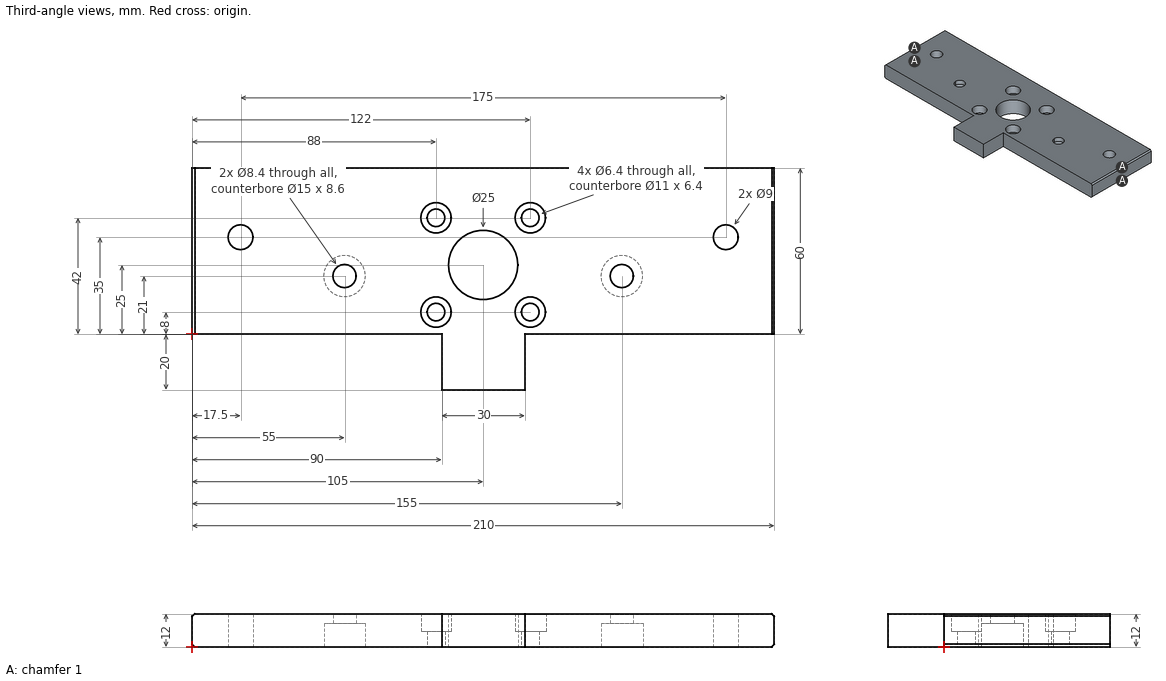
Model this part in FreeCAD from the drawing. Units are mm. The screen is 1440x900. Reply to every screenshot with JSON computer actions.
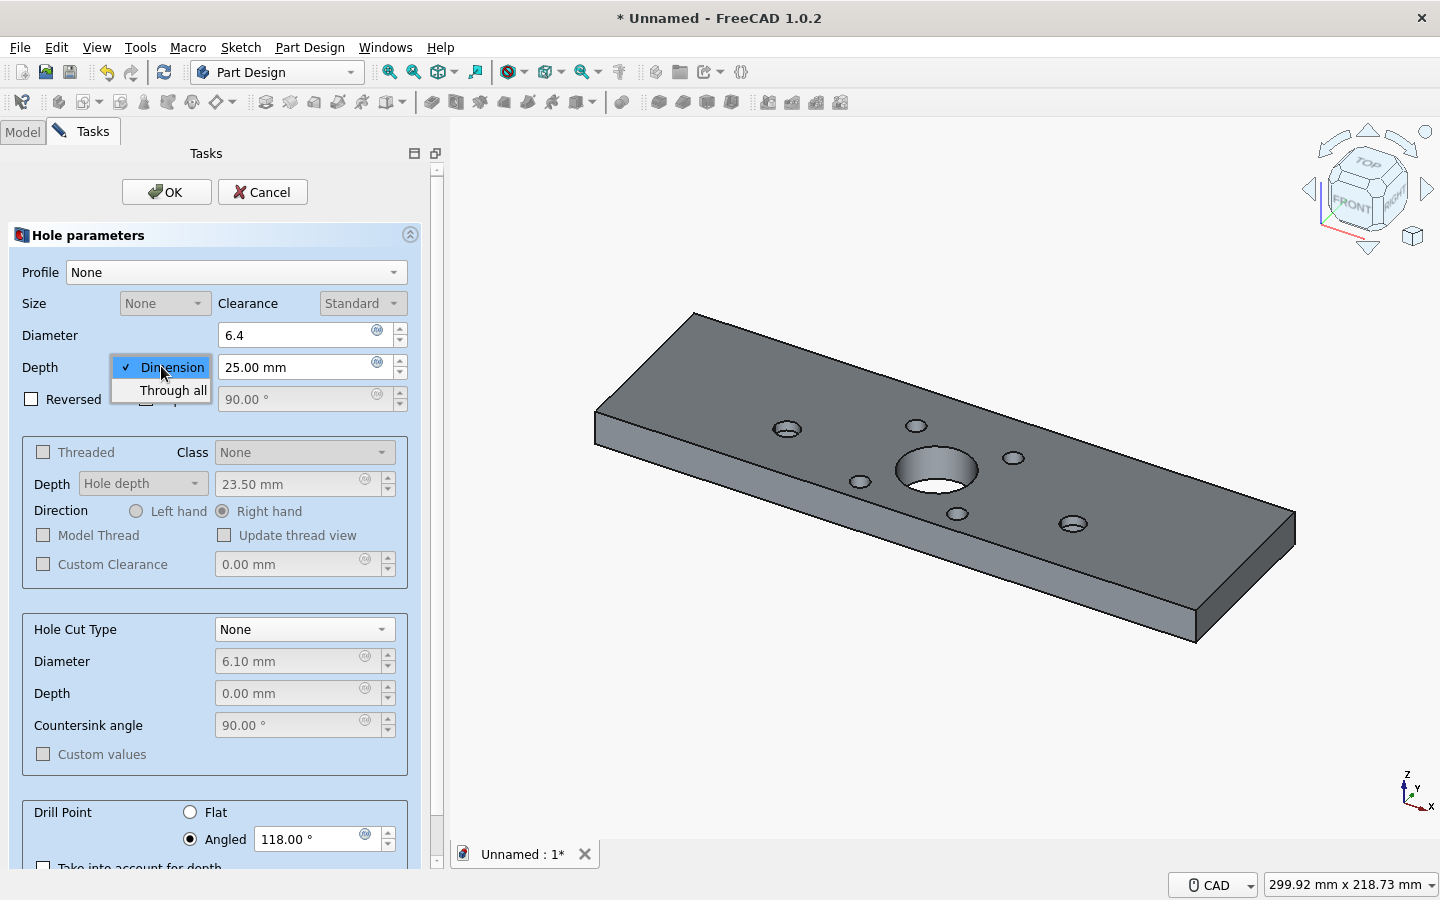
{"action": "left_click", "coordinate": [160, 390]}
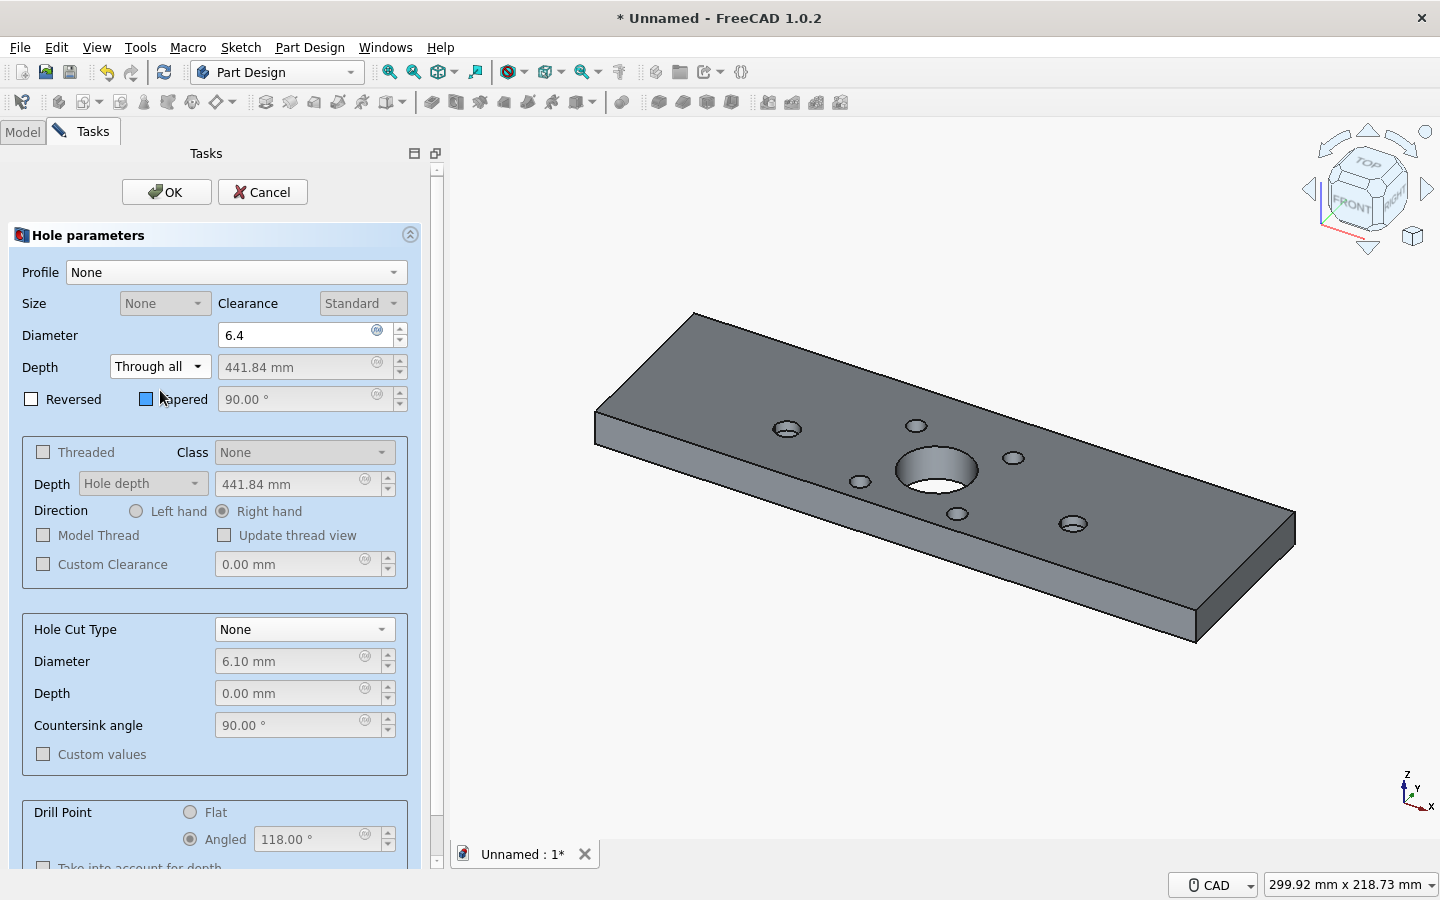
{"action": "left_click", "coordinate": [306, 630]}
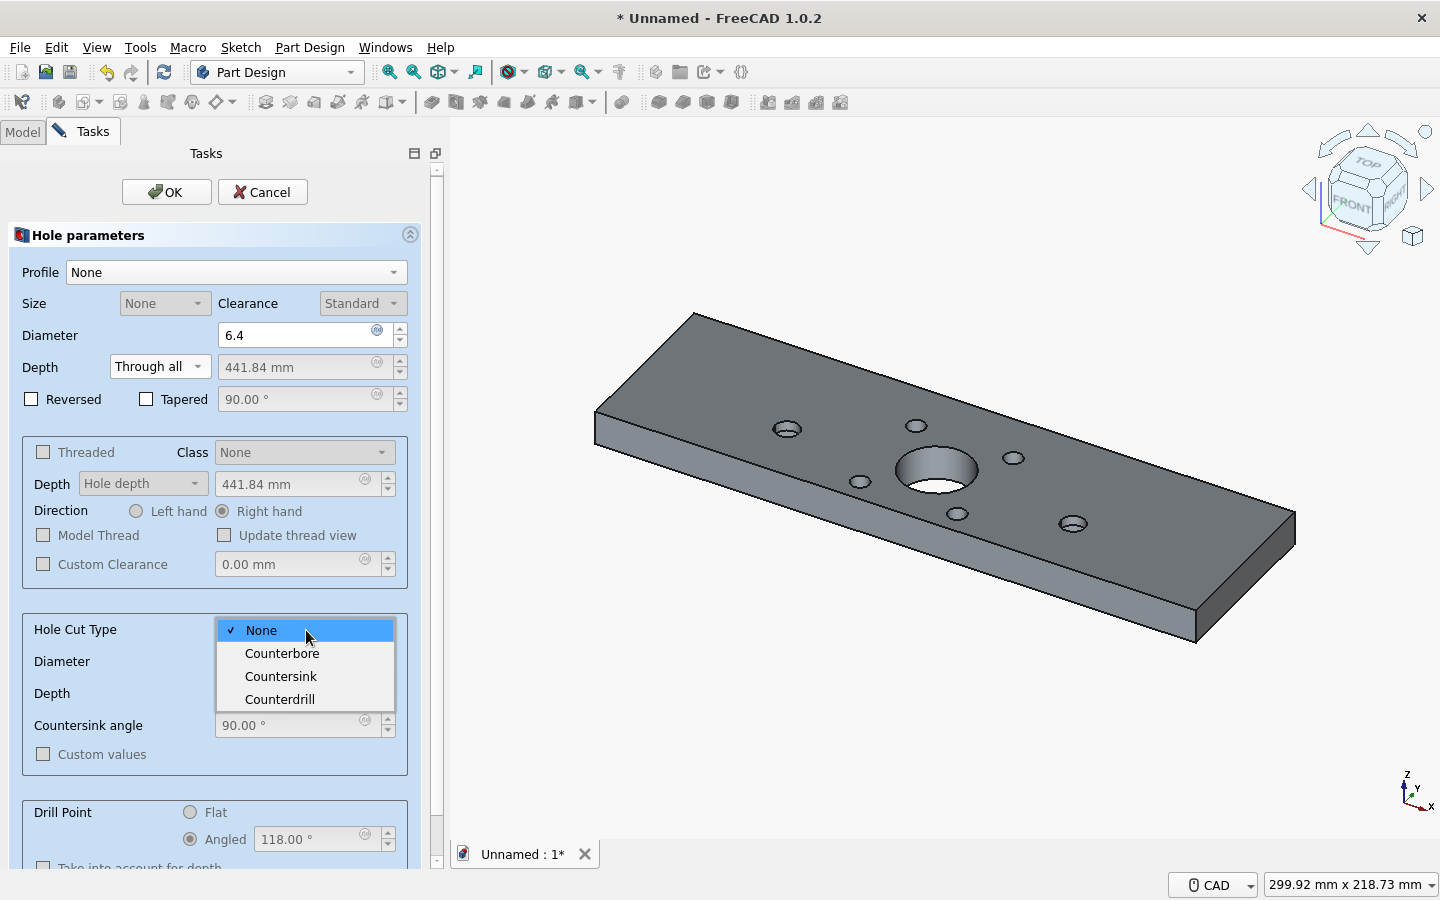
{"action": "left_click", "coordinate": [304, 654]}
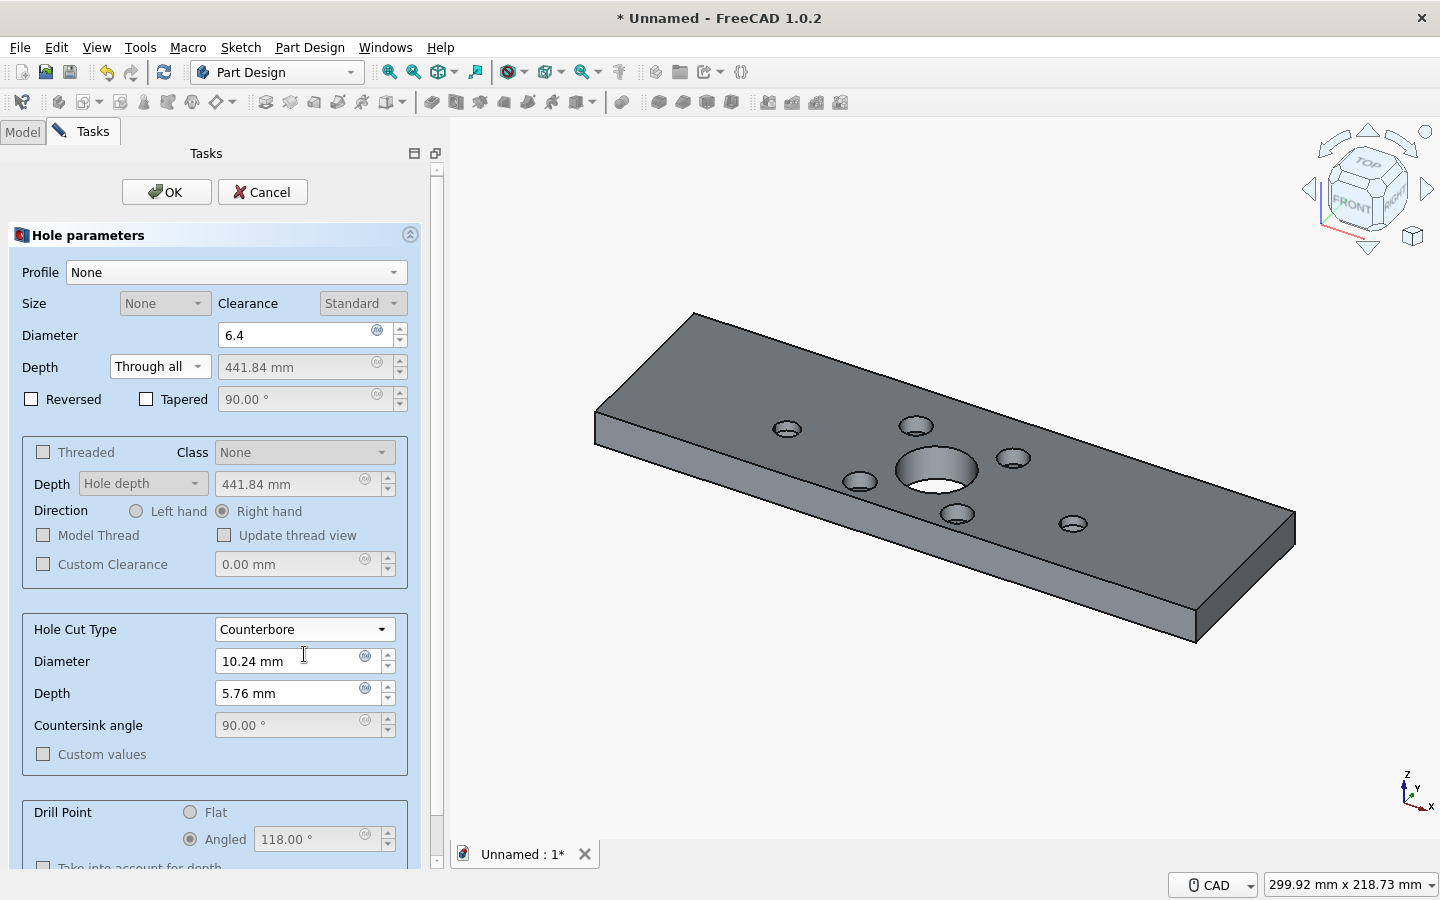
{"action": "triple_click", "coordinate": [298, 661]}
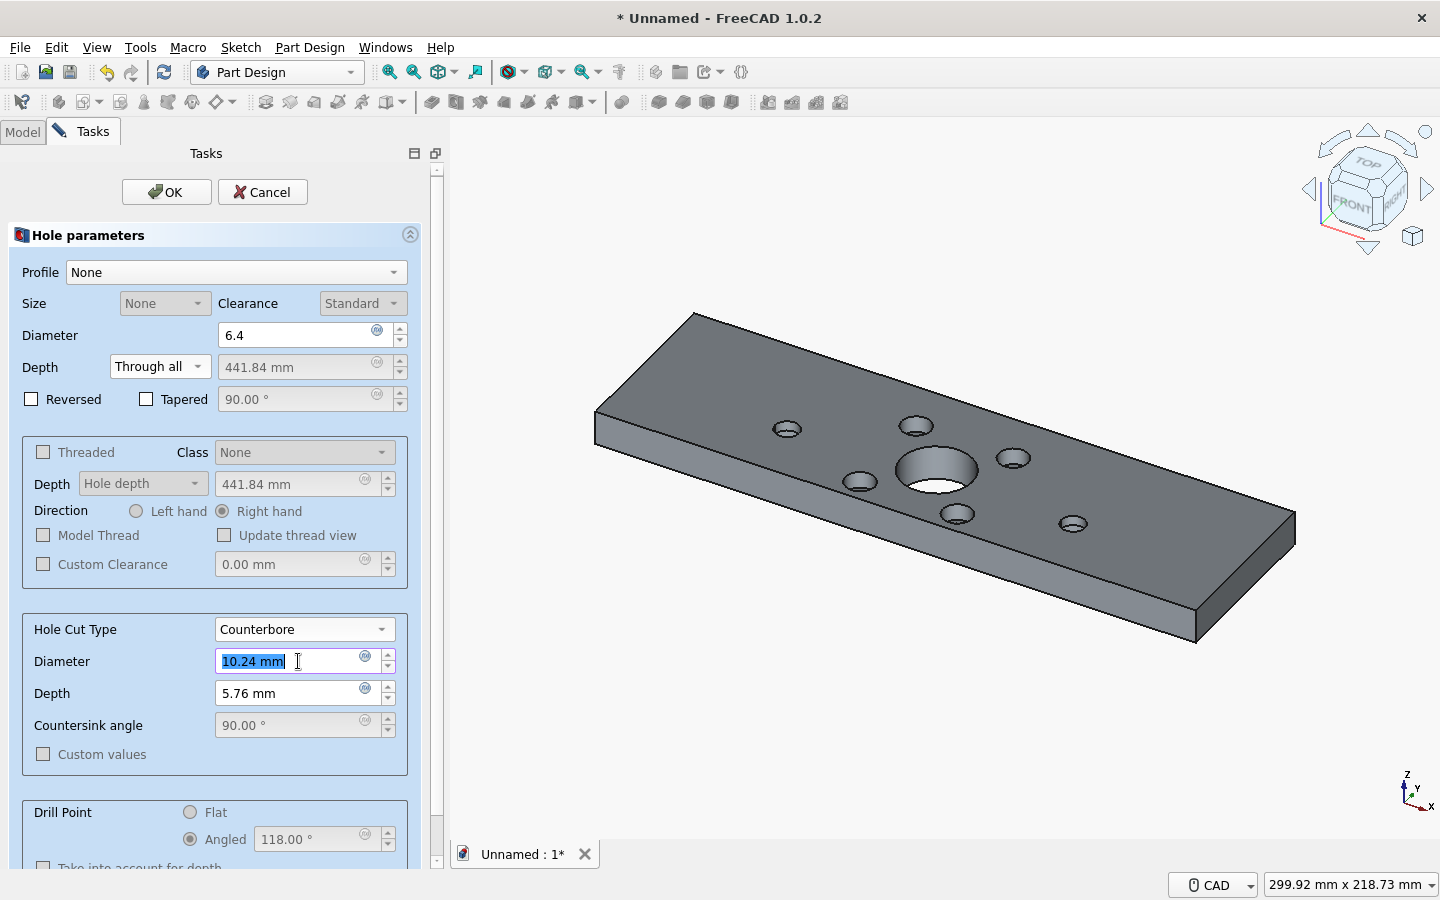
{"action": "type", "text": "11"}
{"action": "key", "text": "Tab"}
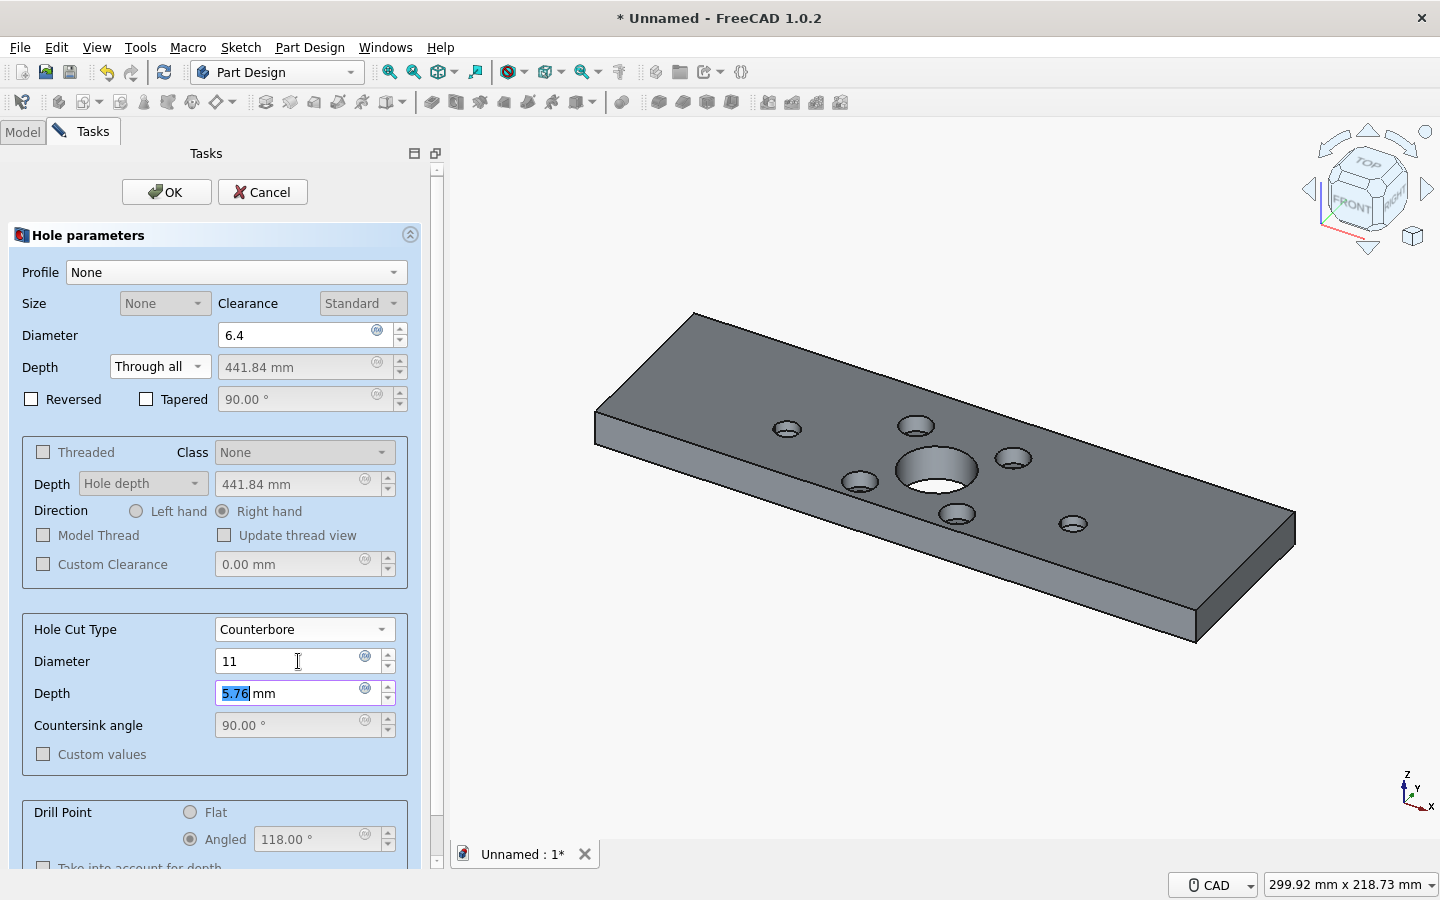
{"action": "type", "text": "6.4"}
{"action": "key", "text": "Tab"}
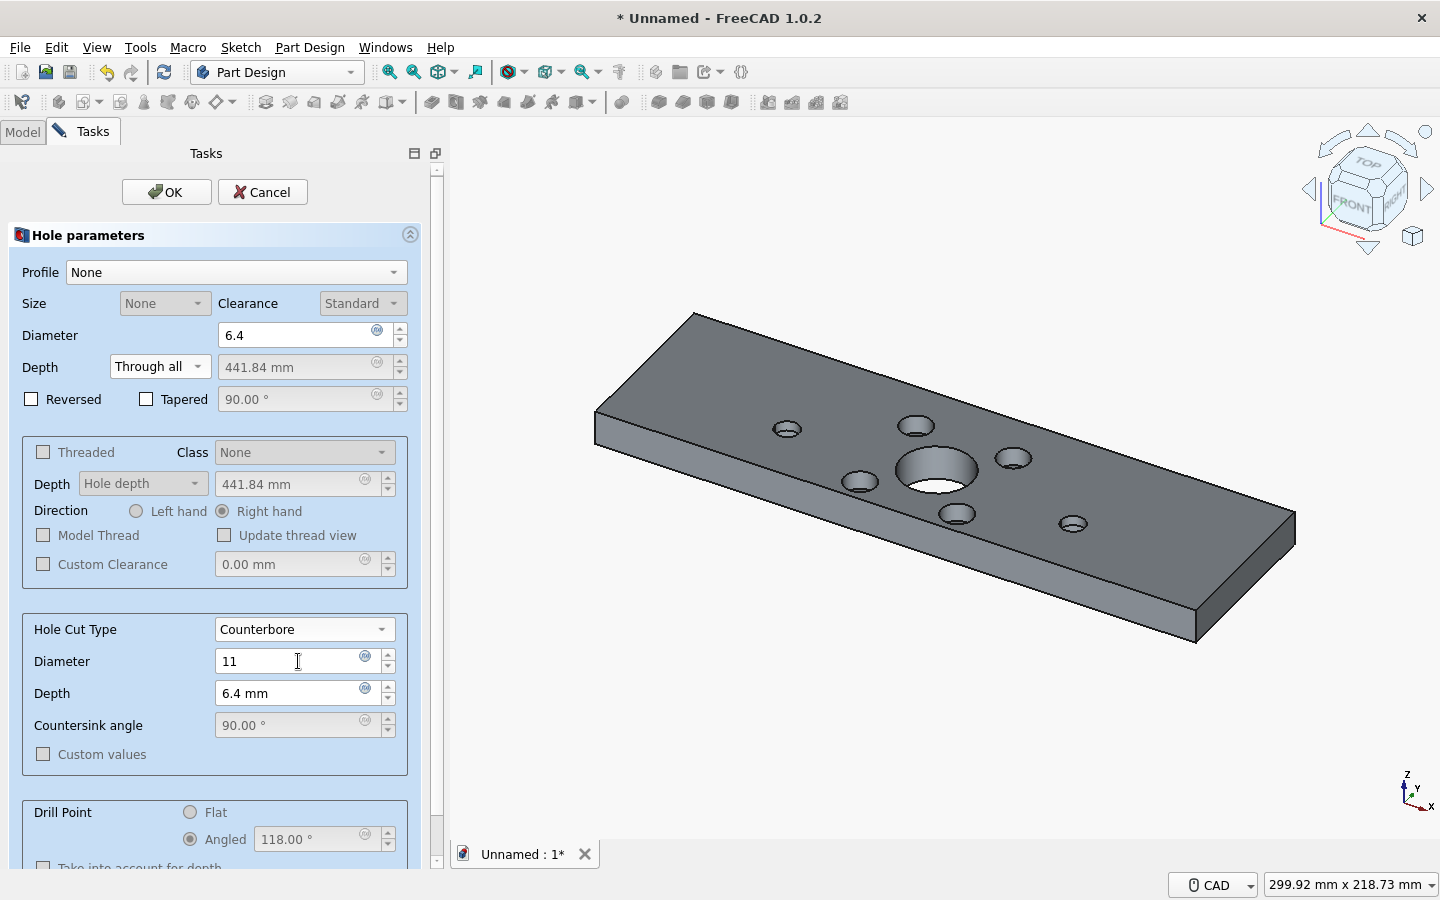
{"action": "left_click", "coordinate": [167, 192]}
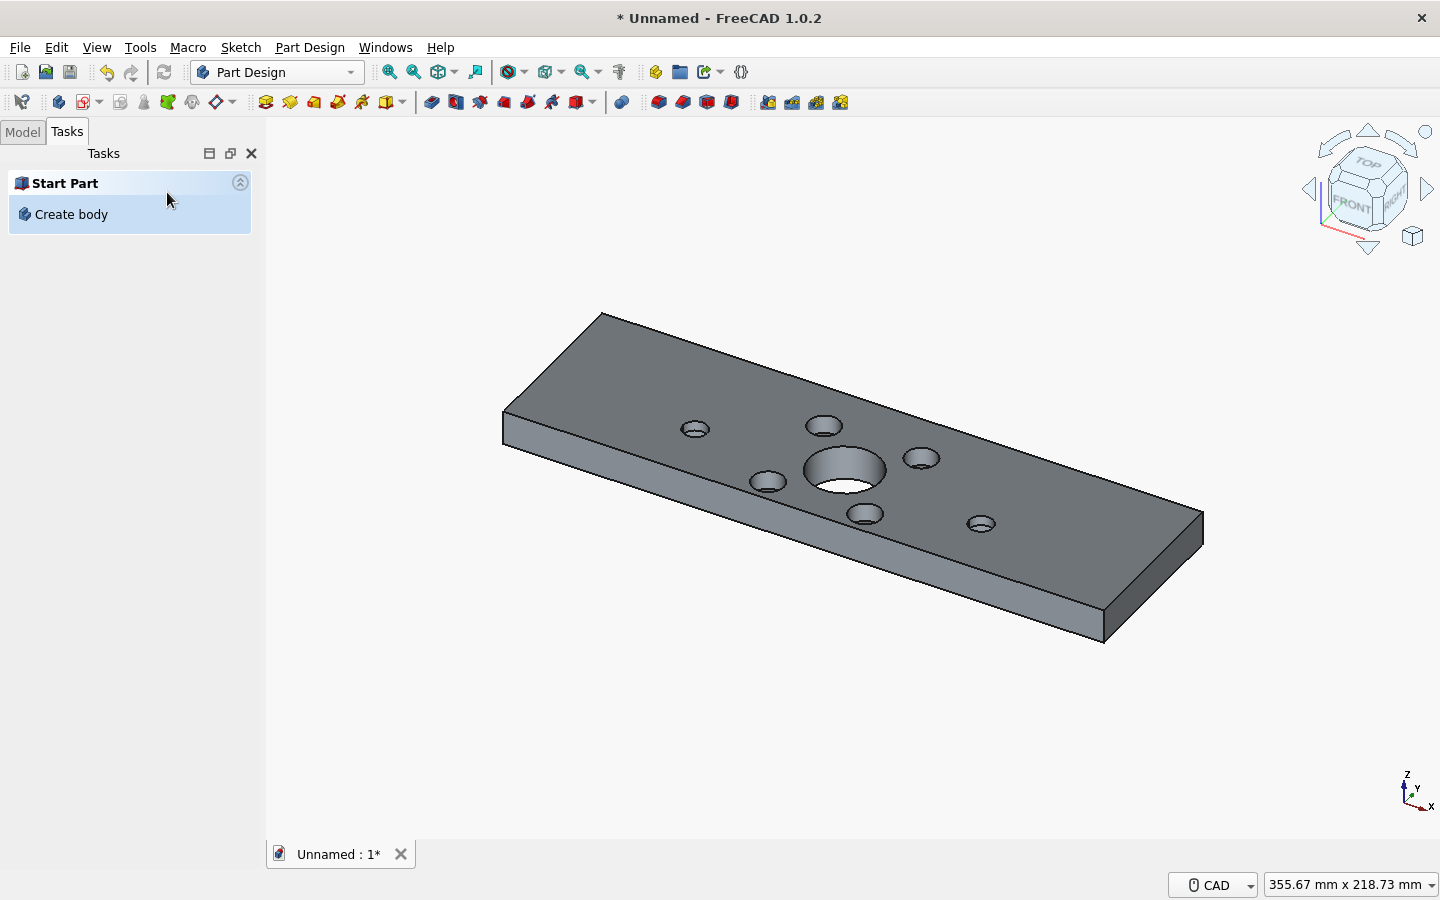
{"action": "left_click", "coordinate": [1153, 560]}